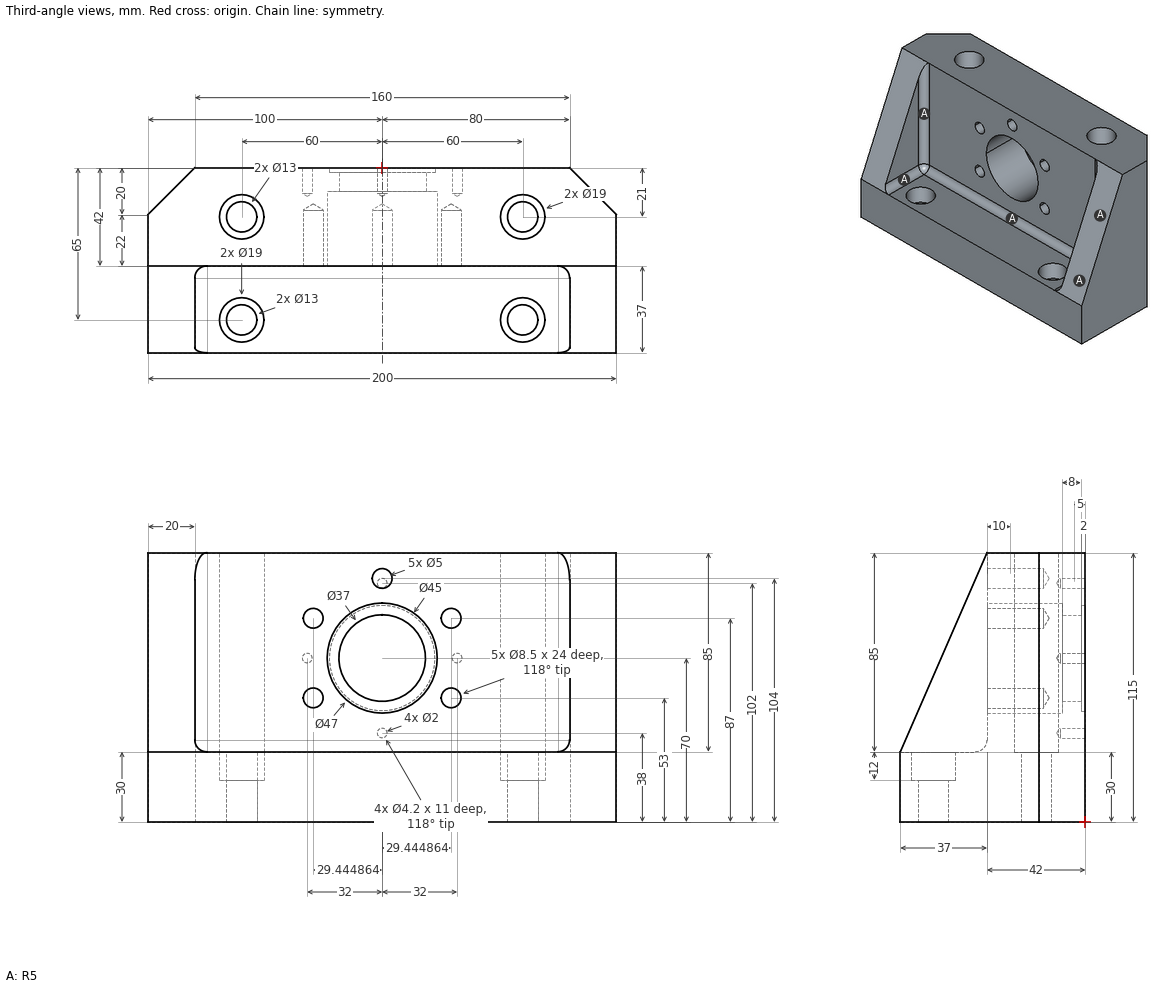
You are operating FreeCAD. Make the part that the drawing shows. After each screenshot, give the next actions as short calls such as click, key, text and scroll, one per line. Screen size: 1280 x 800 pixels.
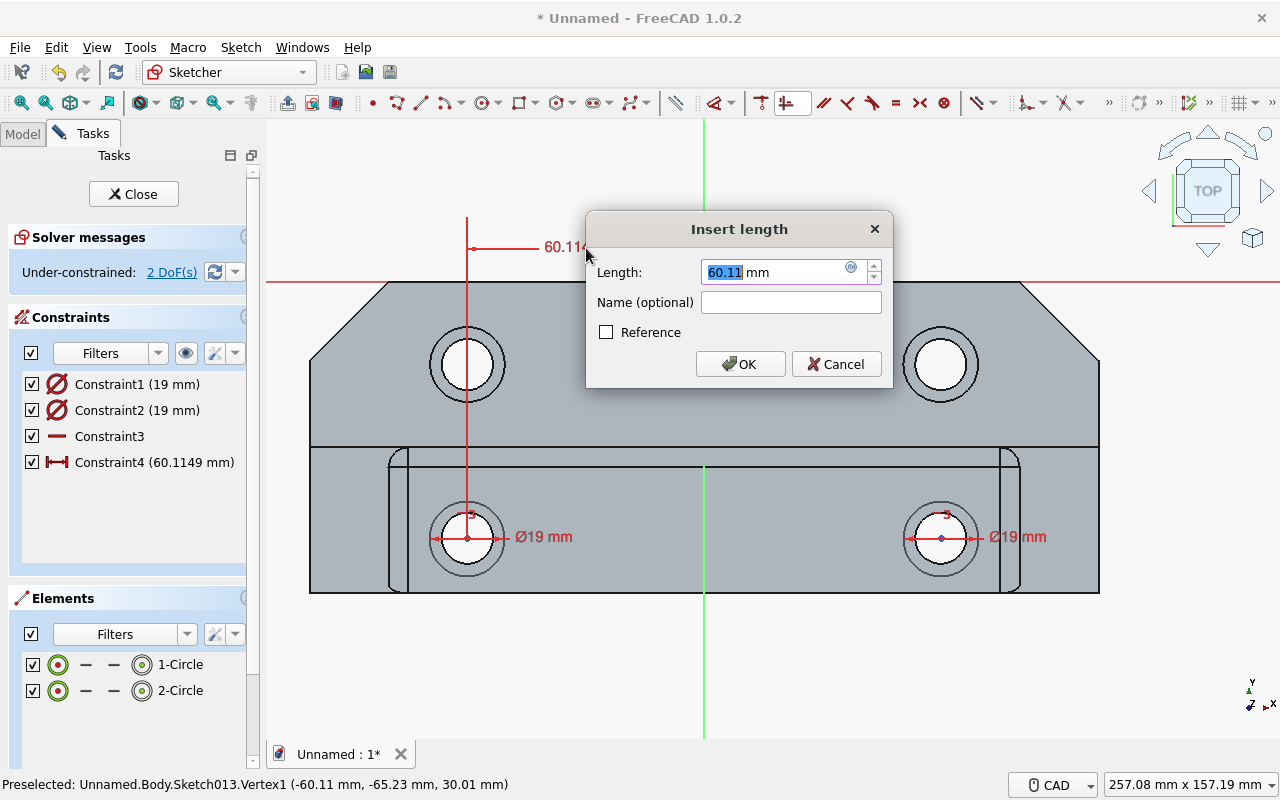
text(60)
key(Return)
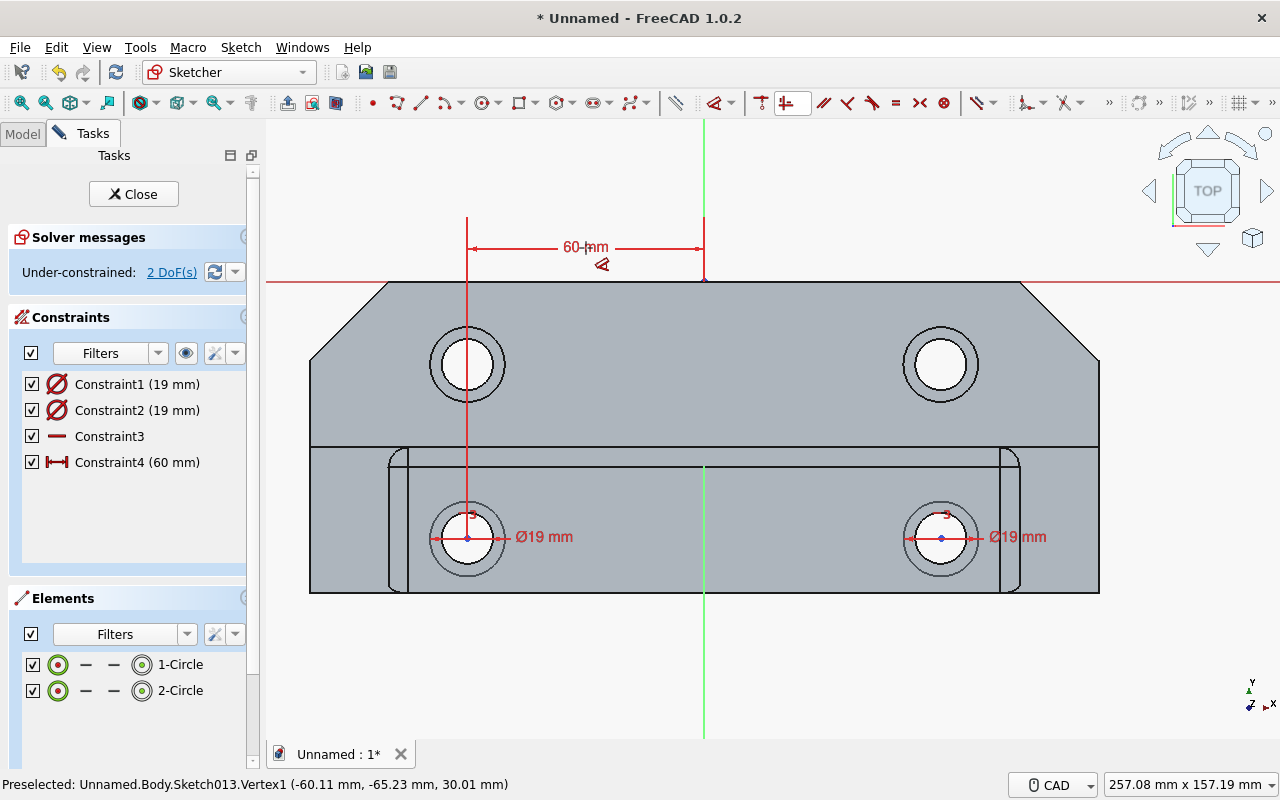
click(467, 539)
click(433, 410)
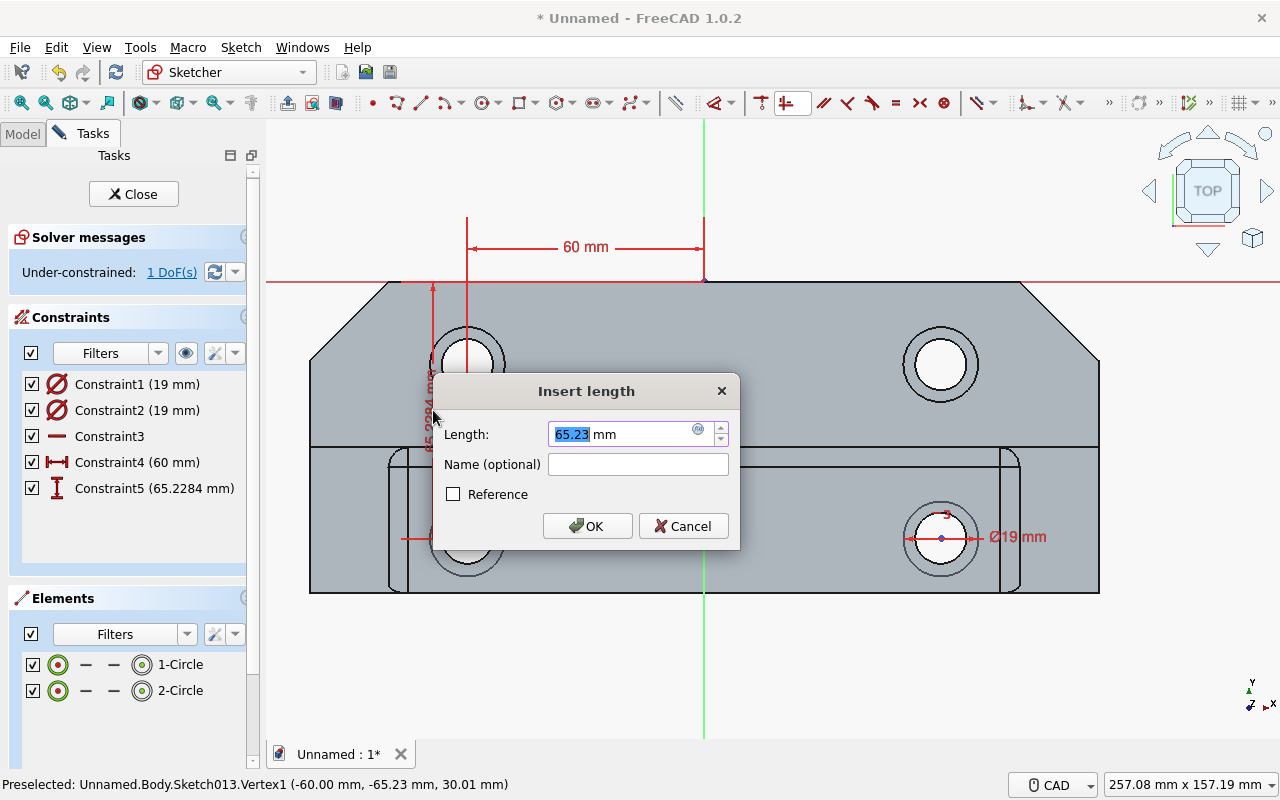
text(65)
key(Return)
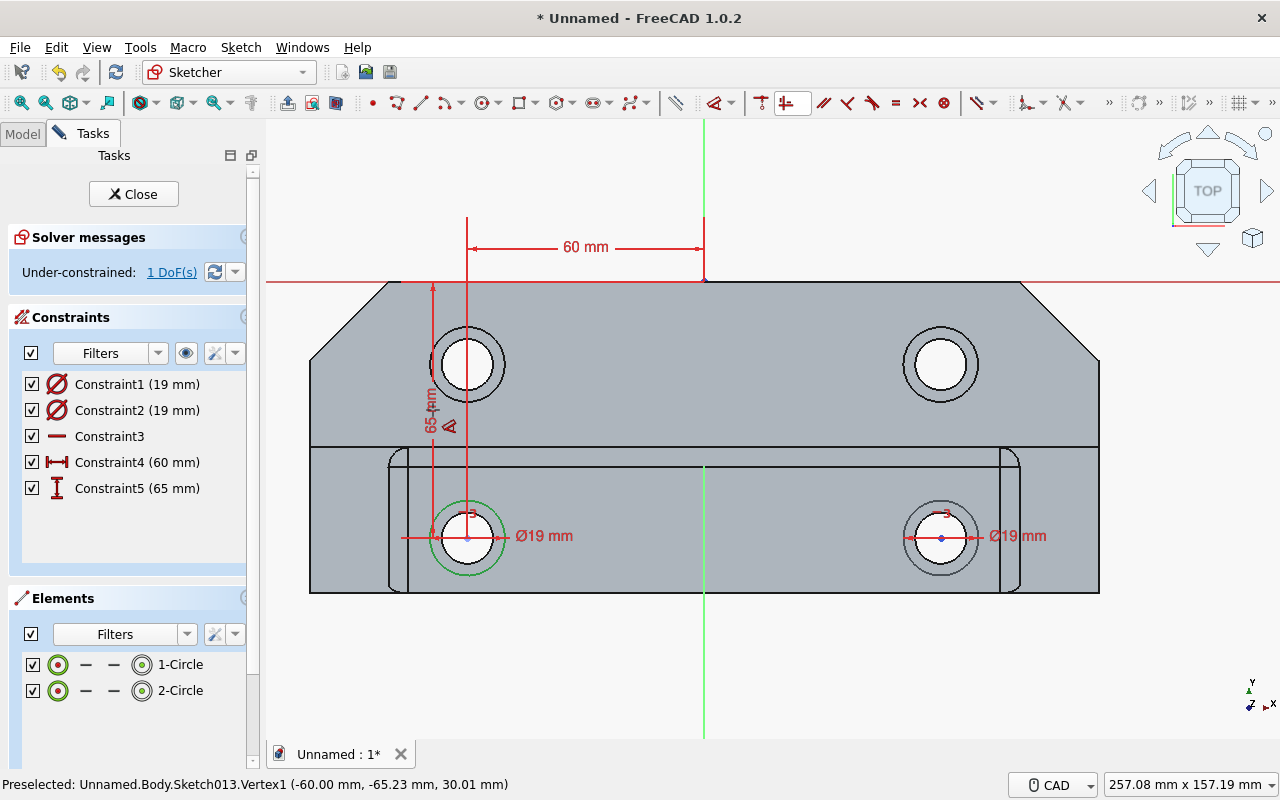
click(941, 538)
click(823, 248)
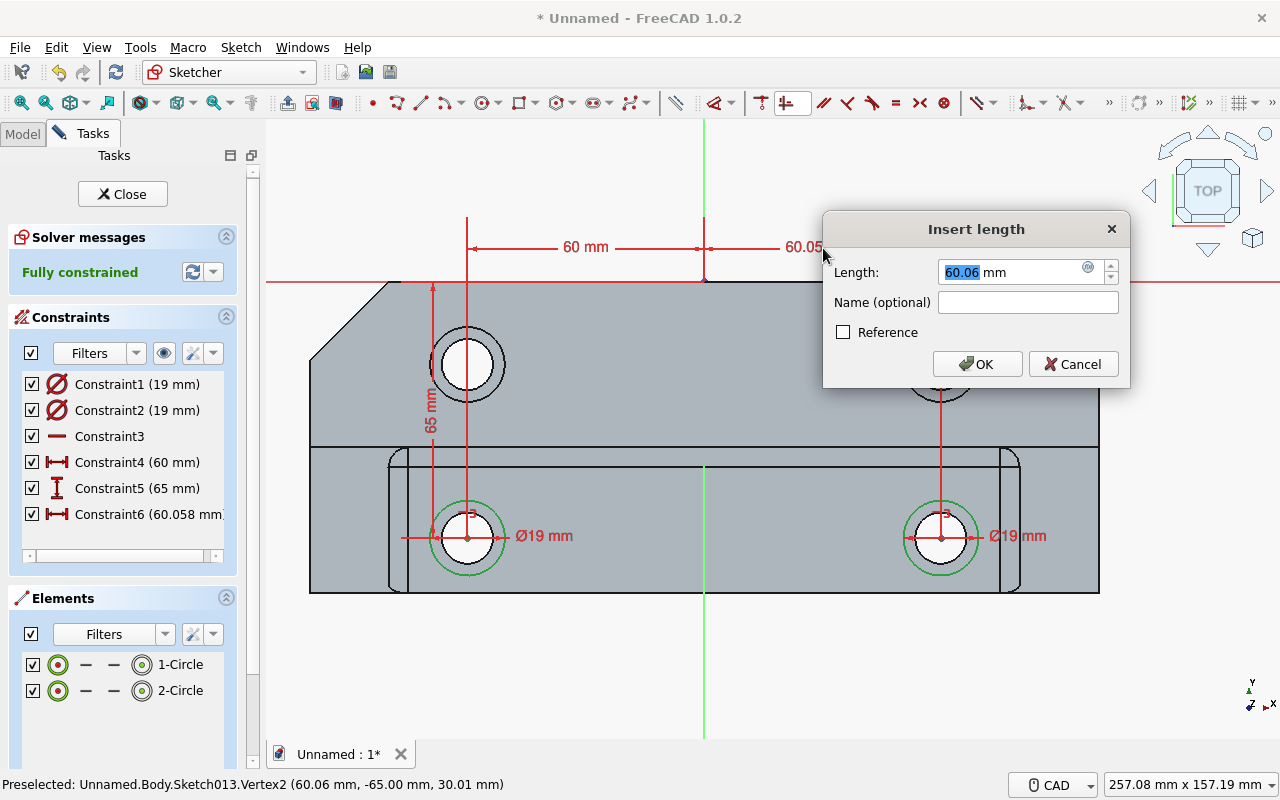
text(60)
key(Return)
key(Escape)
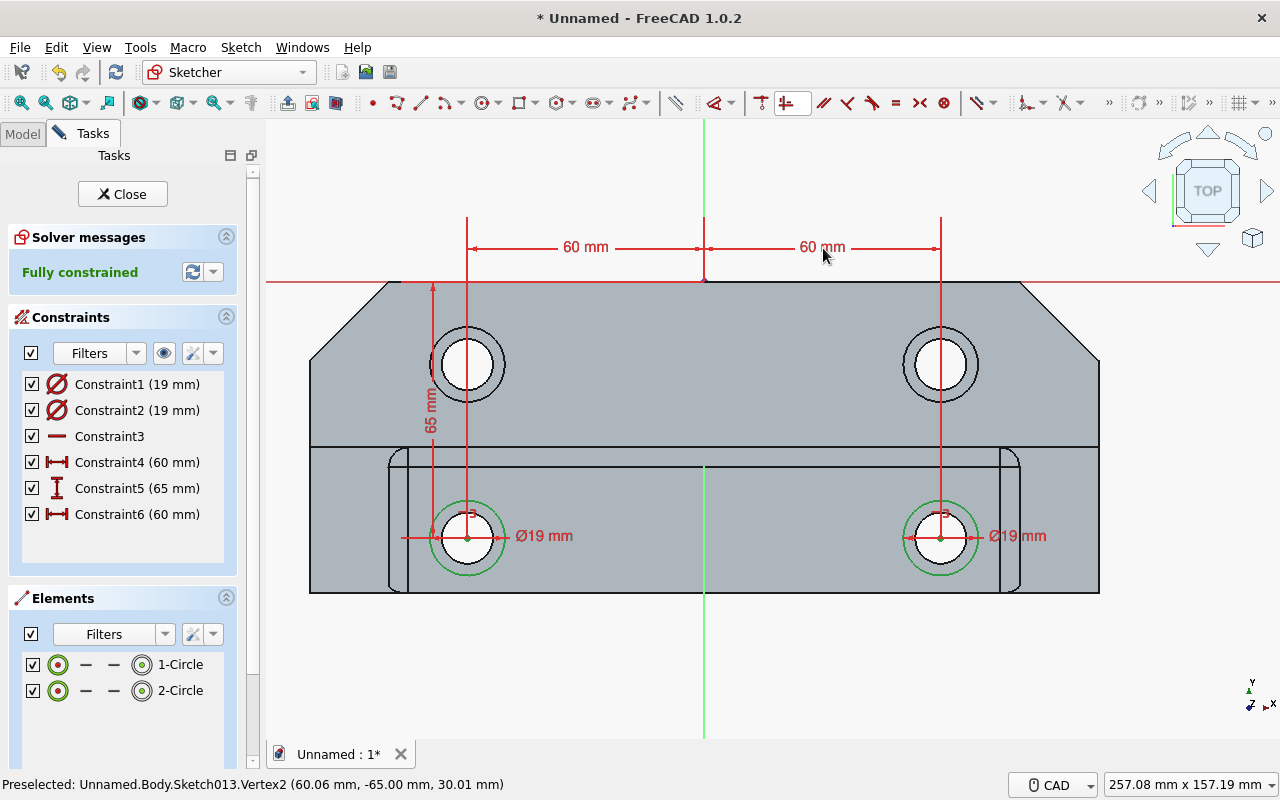
click(123, 194)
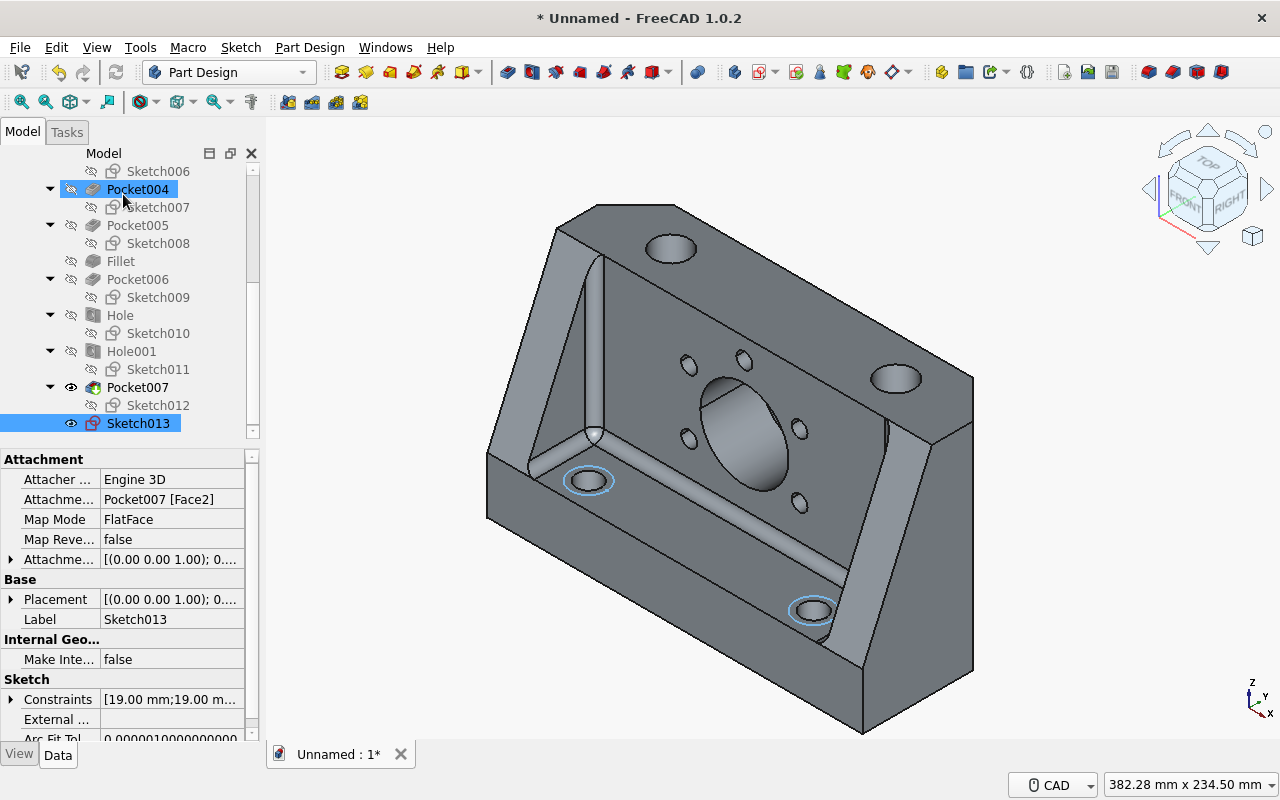
click(508, 72)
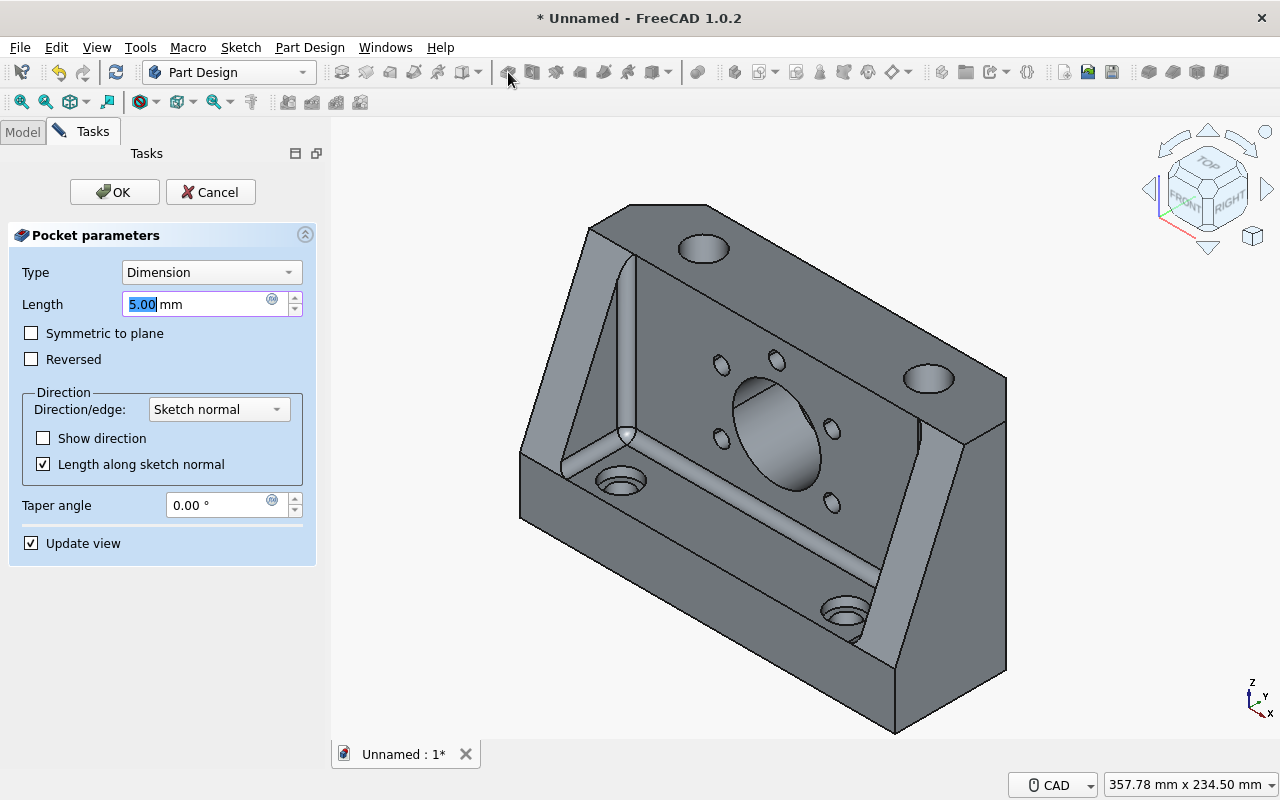
text(12)
key(Tab)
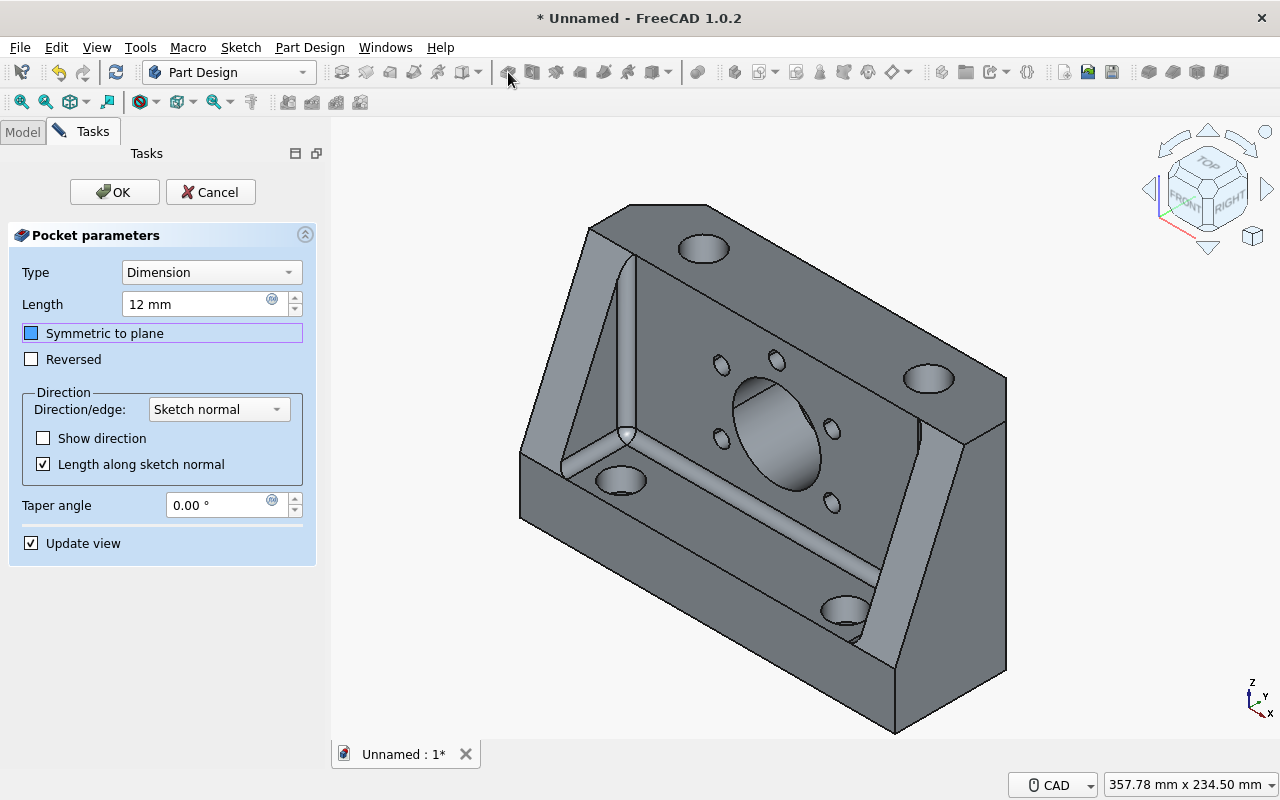
click(115, 192)